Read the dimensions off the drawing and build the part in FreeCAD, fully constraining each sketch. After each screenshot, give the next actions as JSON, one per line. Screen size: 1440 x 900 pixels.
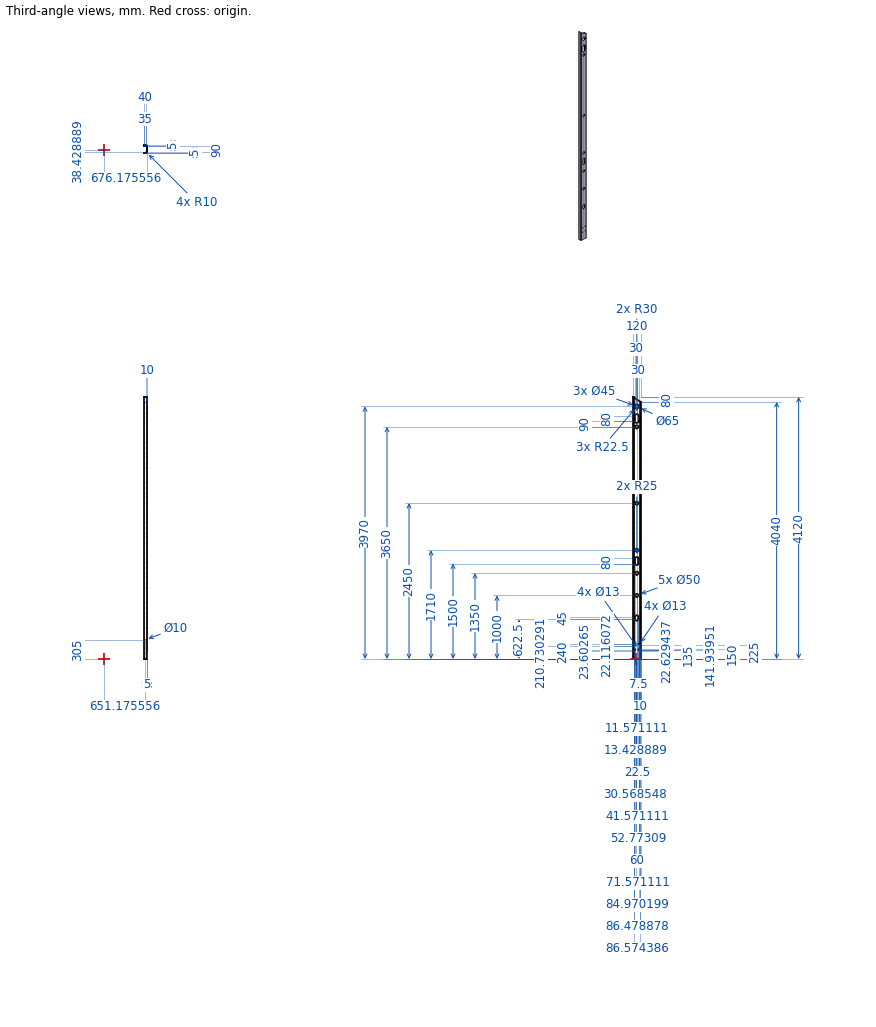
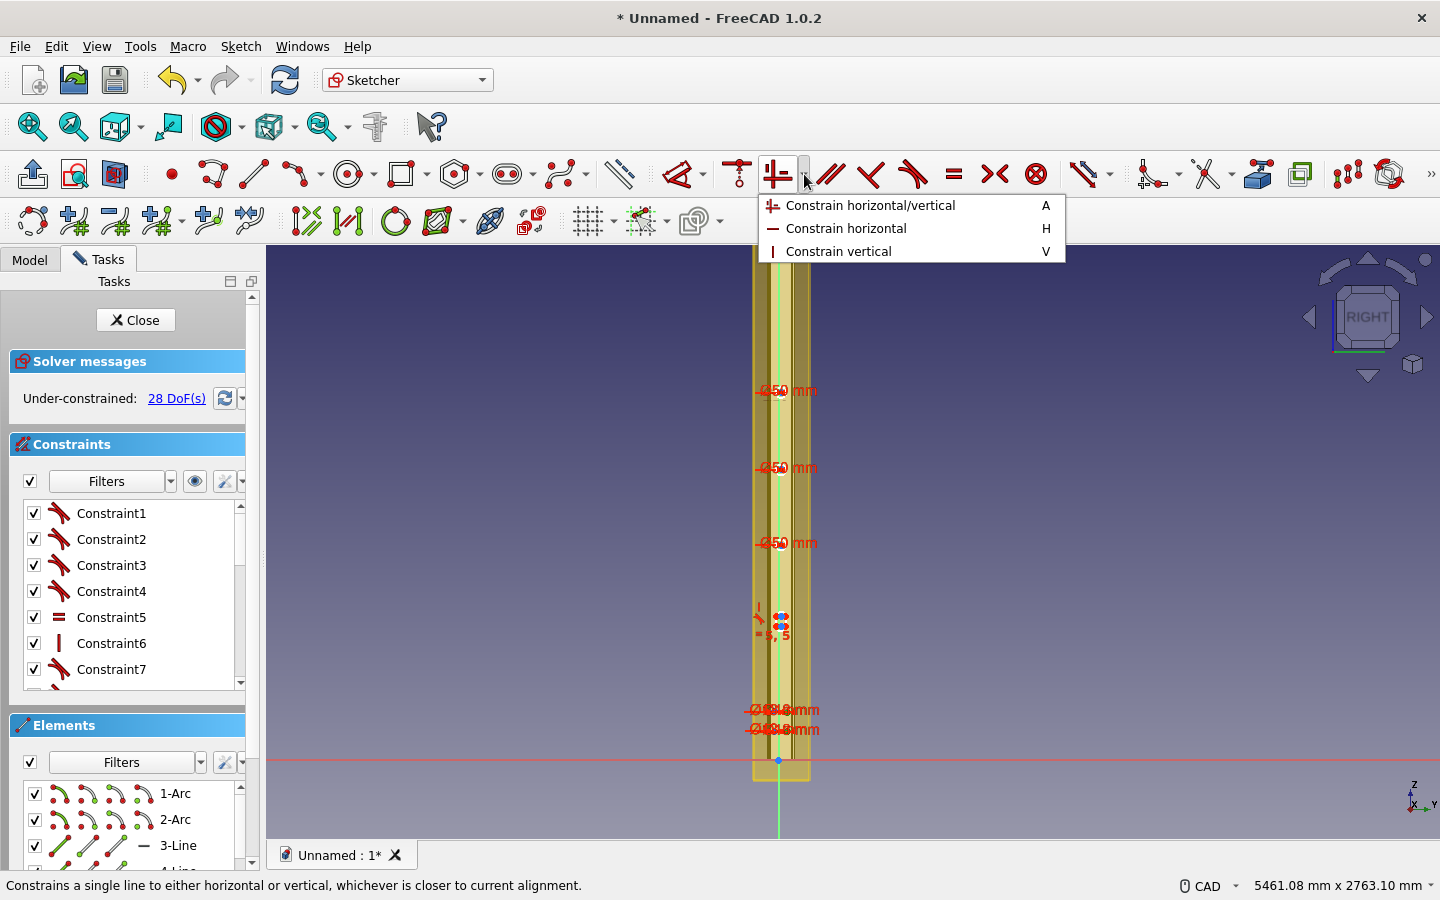
{"action": "left_click", "coordinate": [912, 252]}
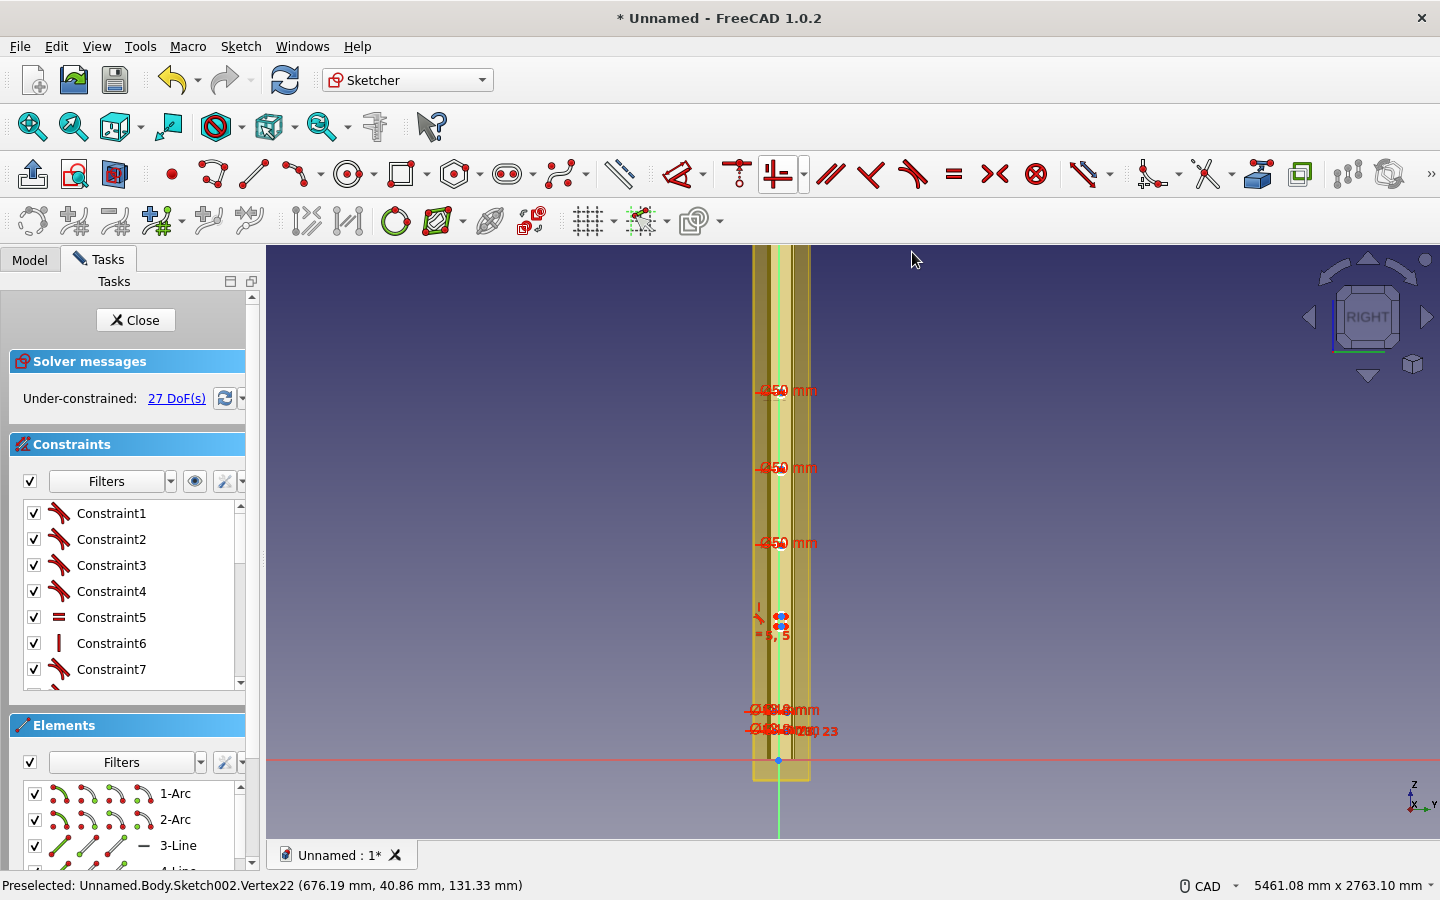
{"action": "scroll", "coordinate": [787, 732], "scroll_direction": "up", "scroll_amount": 4}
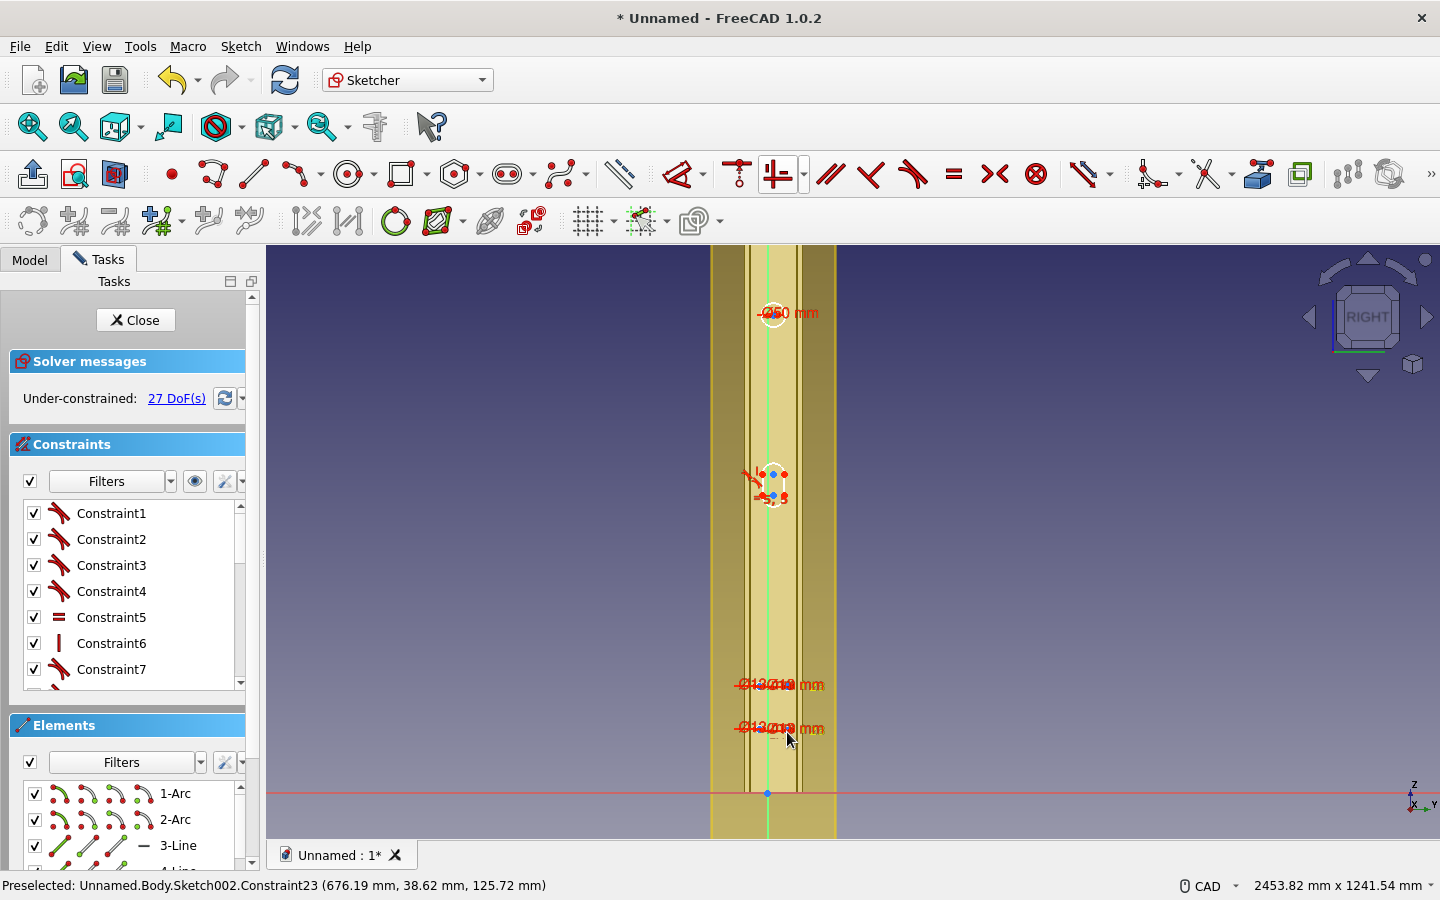
{"action": "left_click", "coordinate": [788, 731]}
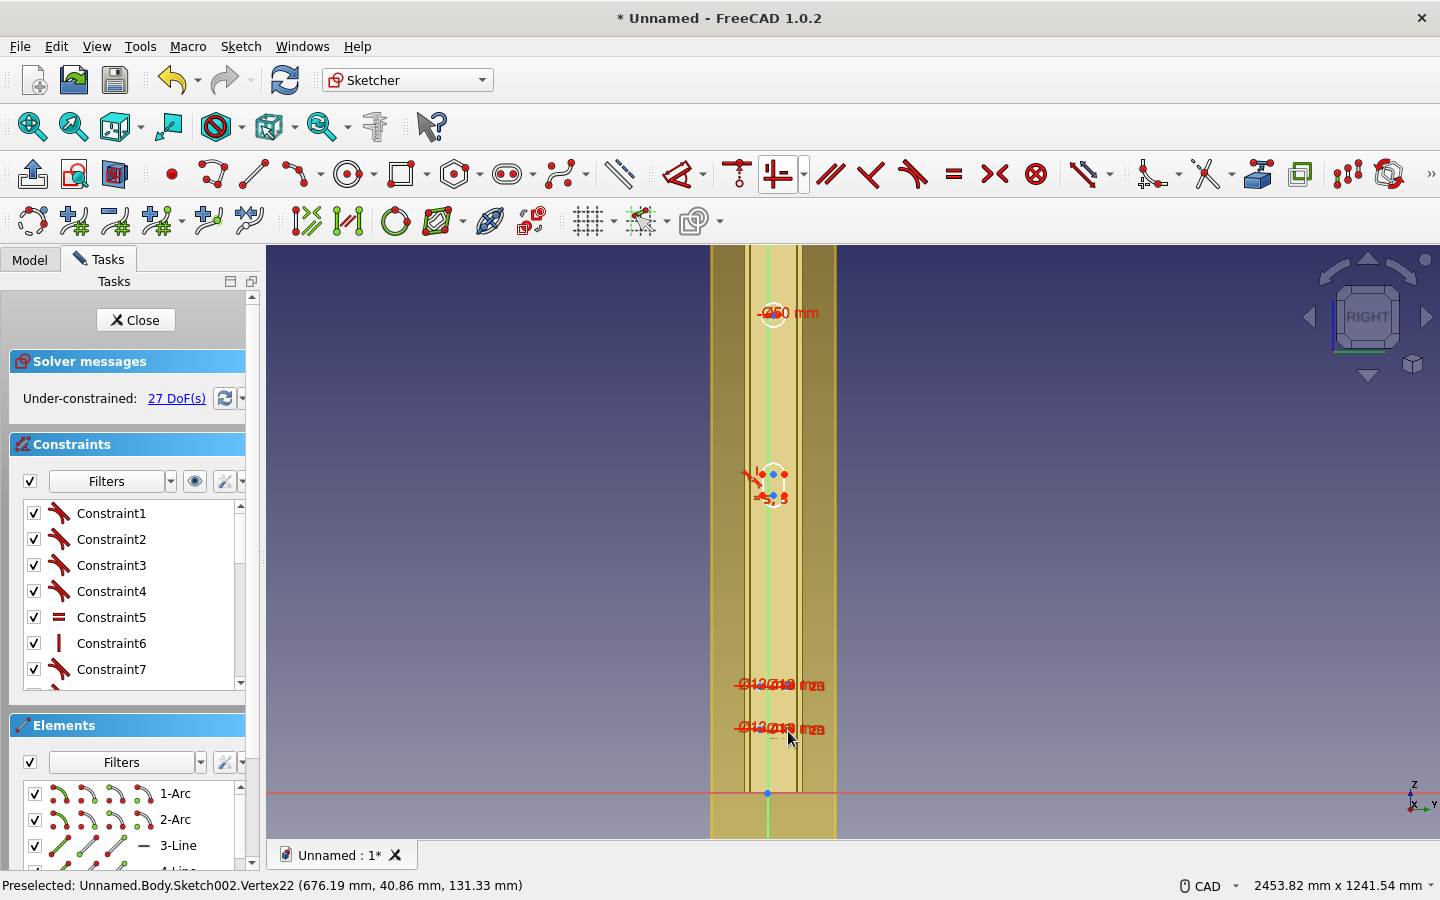
{"action": "left_click", "coordinate": [759, 729]}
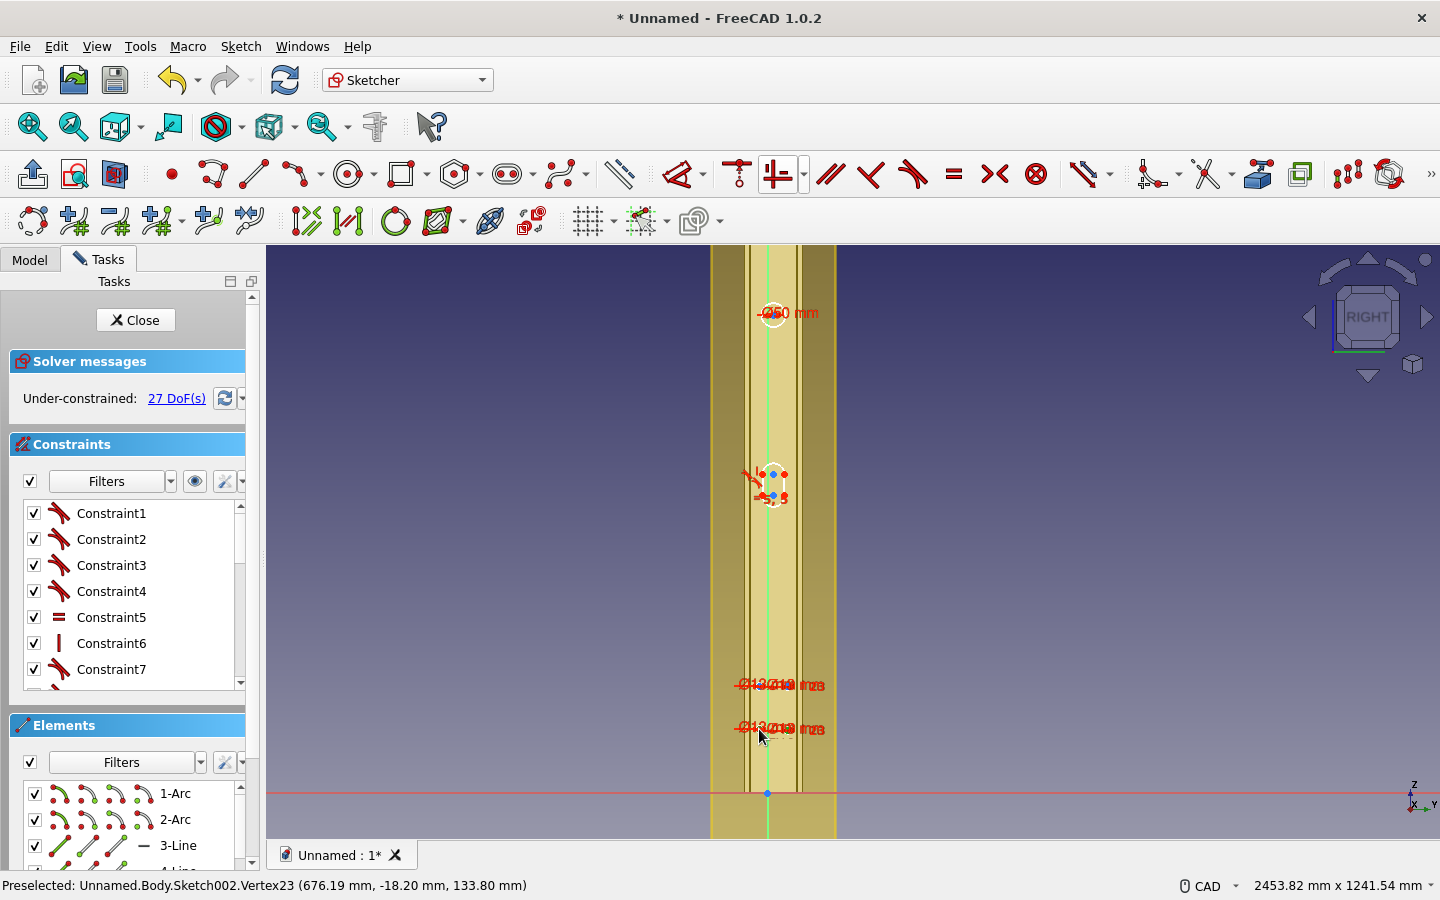
{"action": "key", "text": "h"}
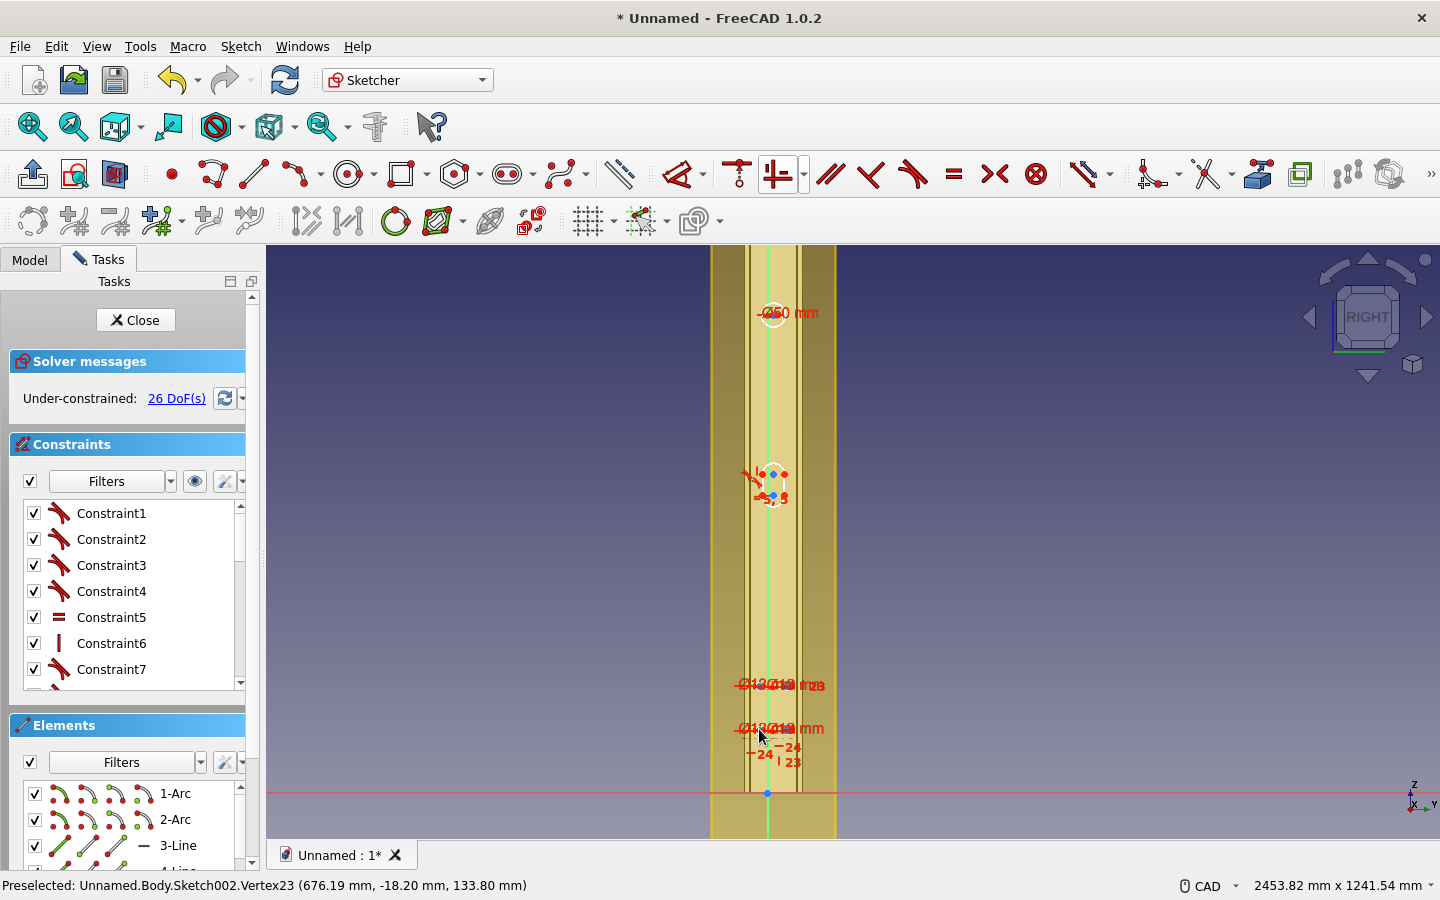
{"action": "left_click", "coordinate": [759, 731]}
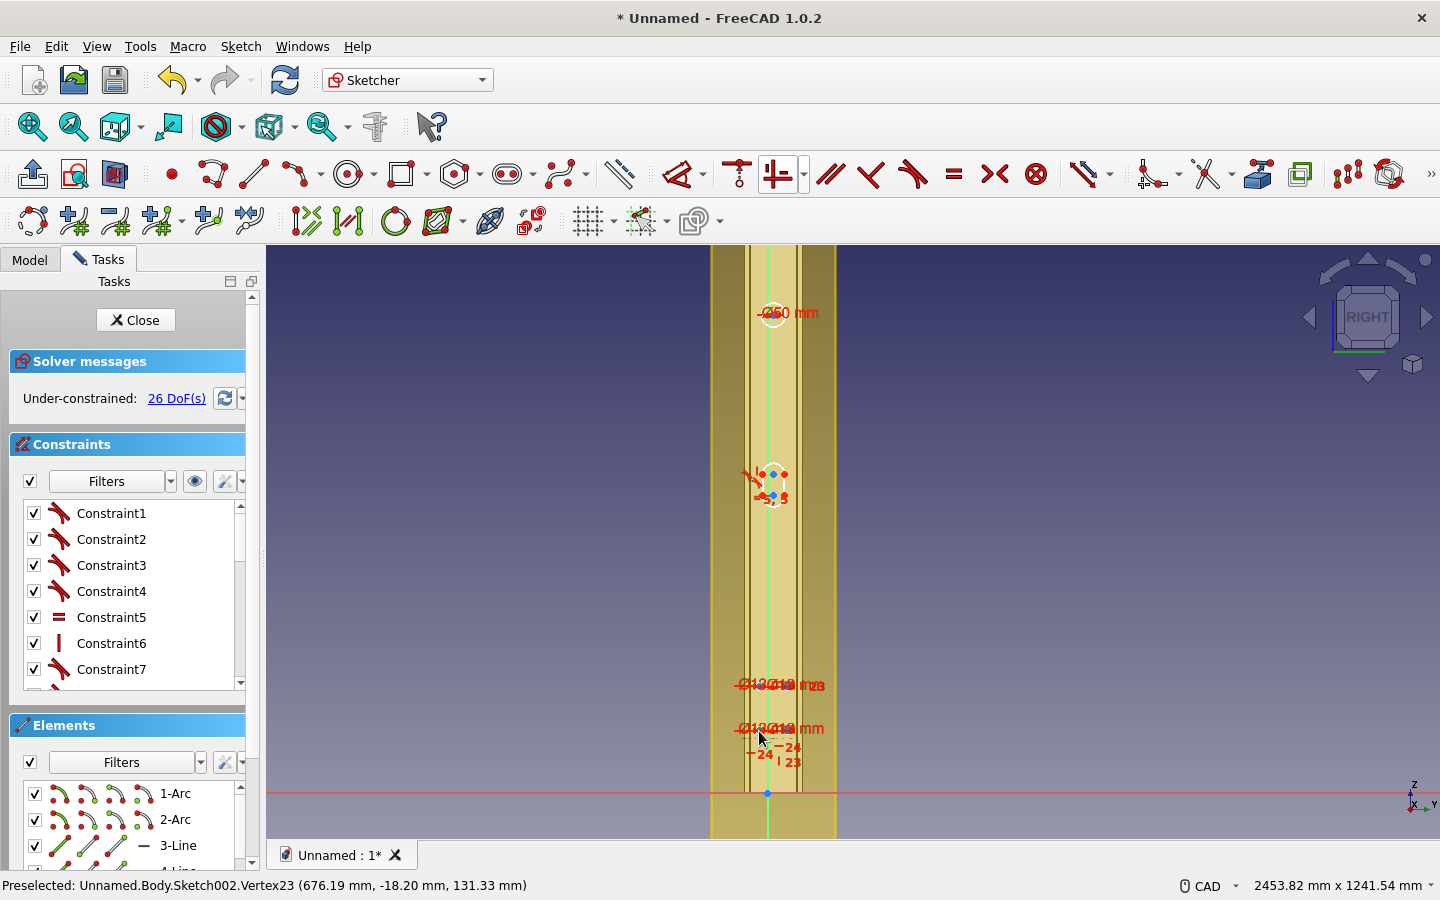
{"action": "left_click", "coordinate": [759, 686]}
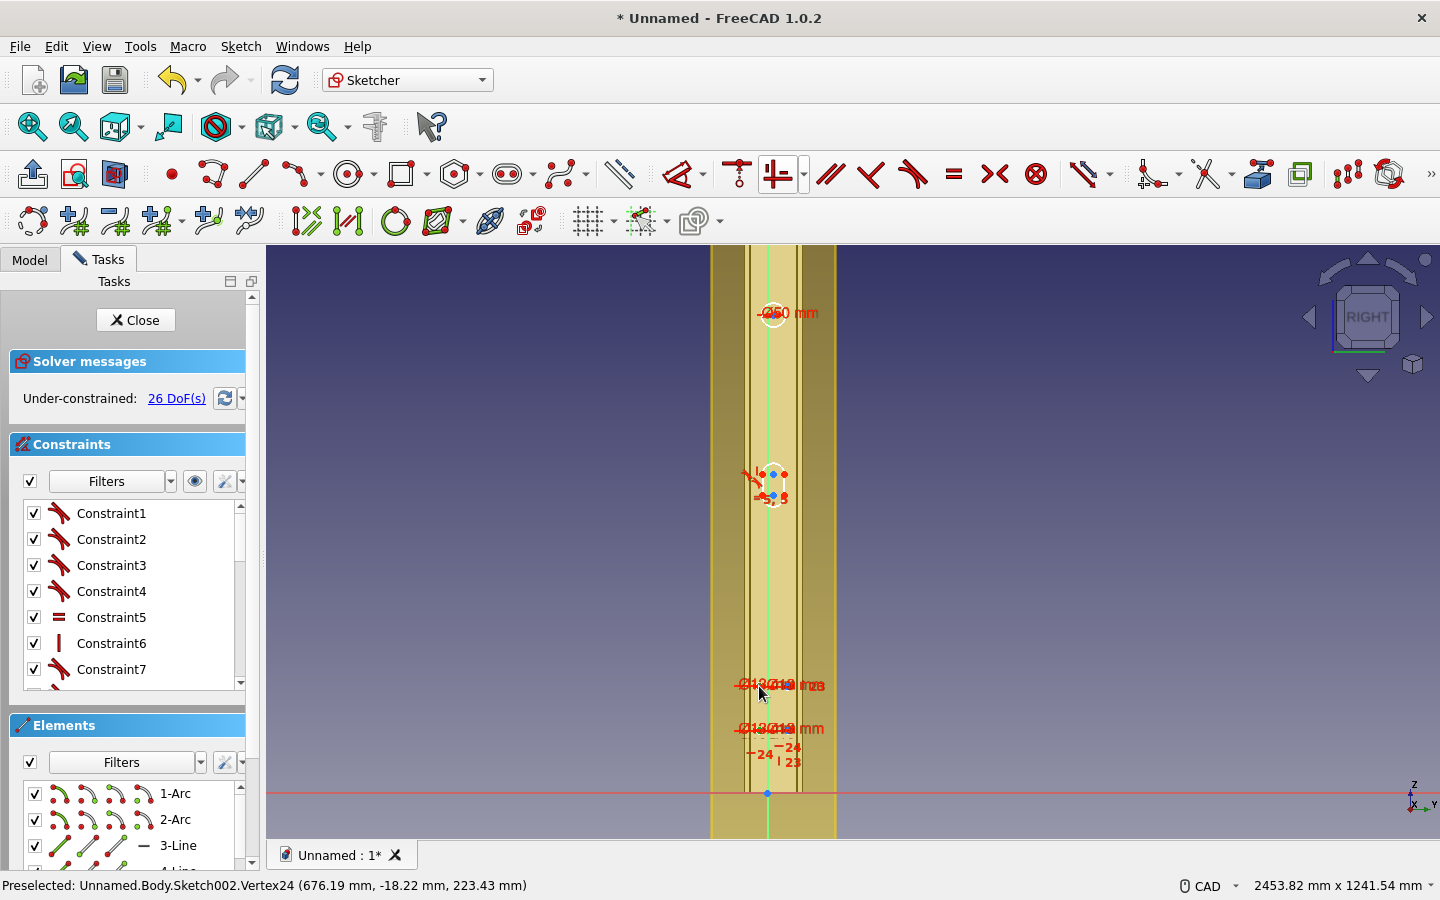
{"action": "left_click", "coordinate": [804, 174]}